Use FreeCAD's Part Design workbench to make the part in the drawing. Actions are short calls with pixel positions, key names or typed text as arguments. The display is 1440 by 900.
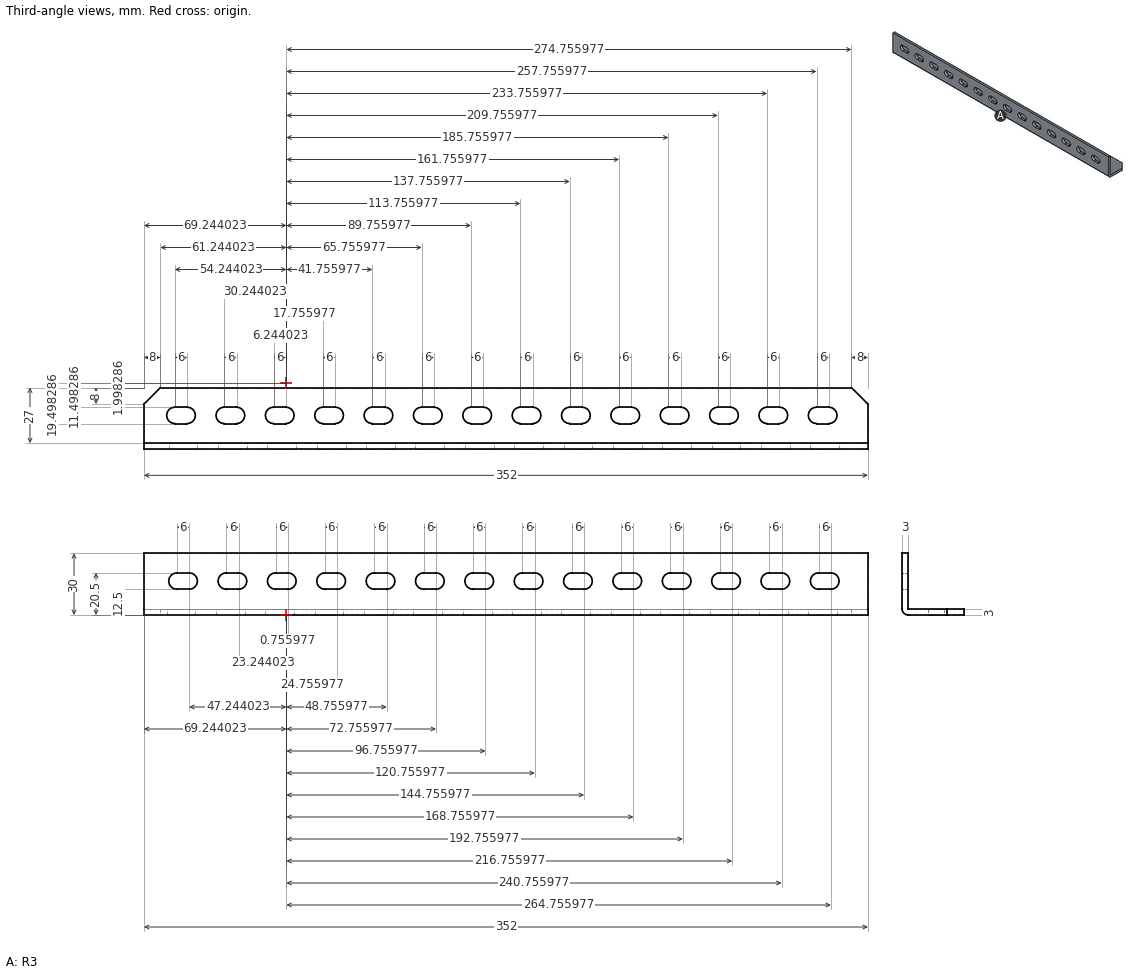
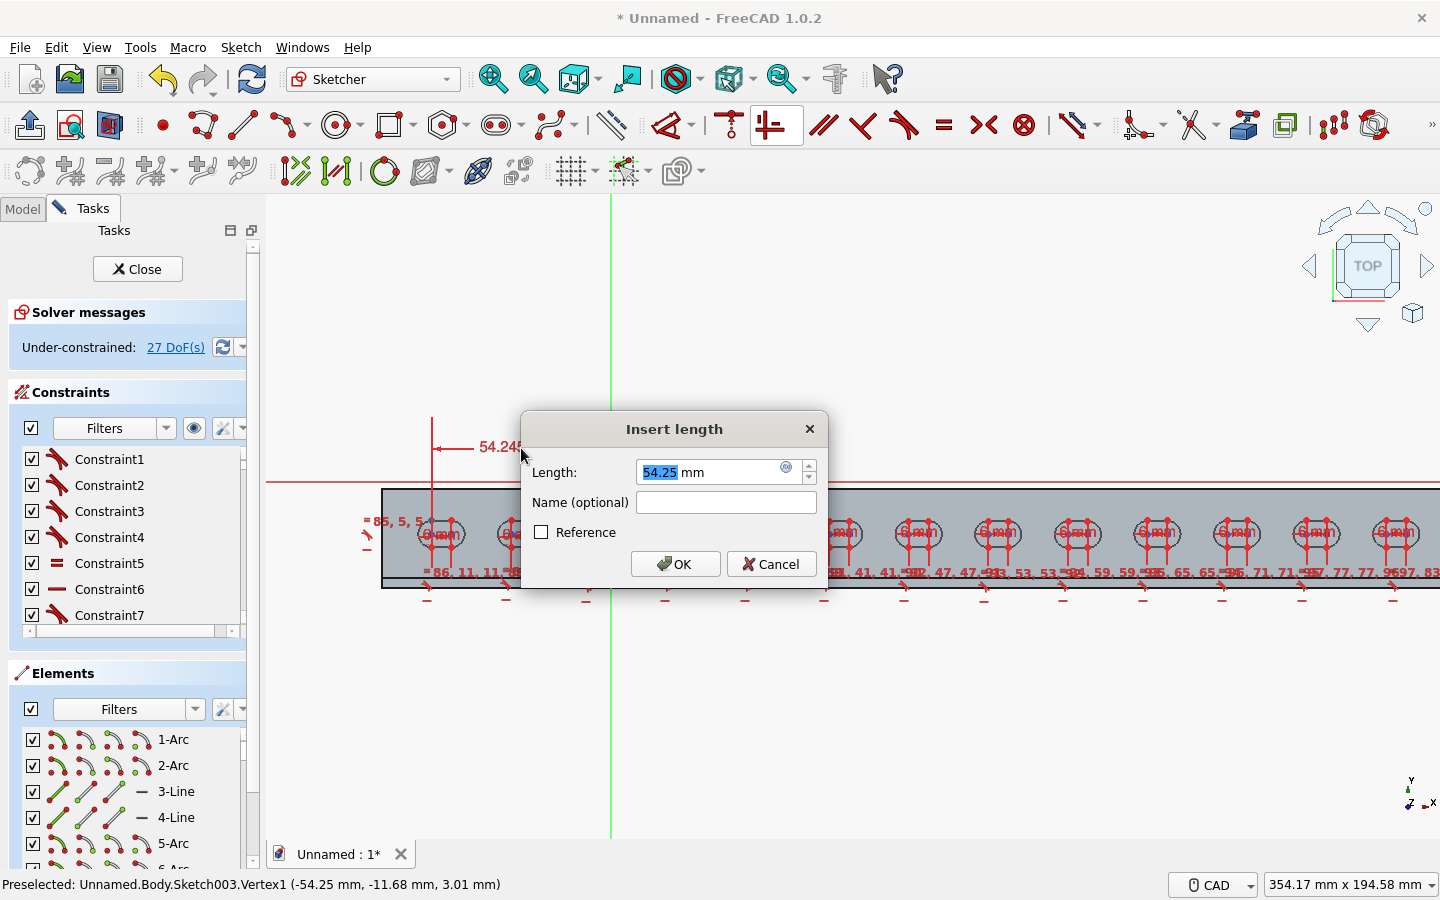
text(54.244023)
key(Return)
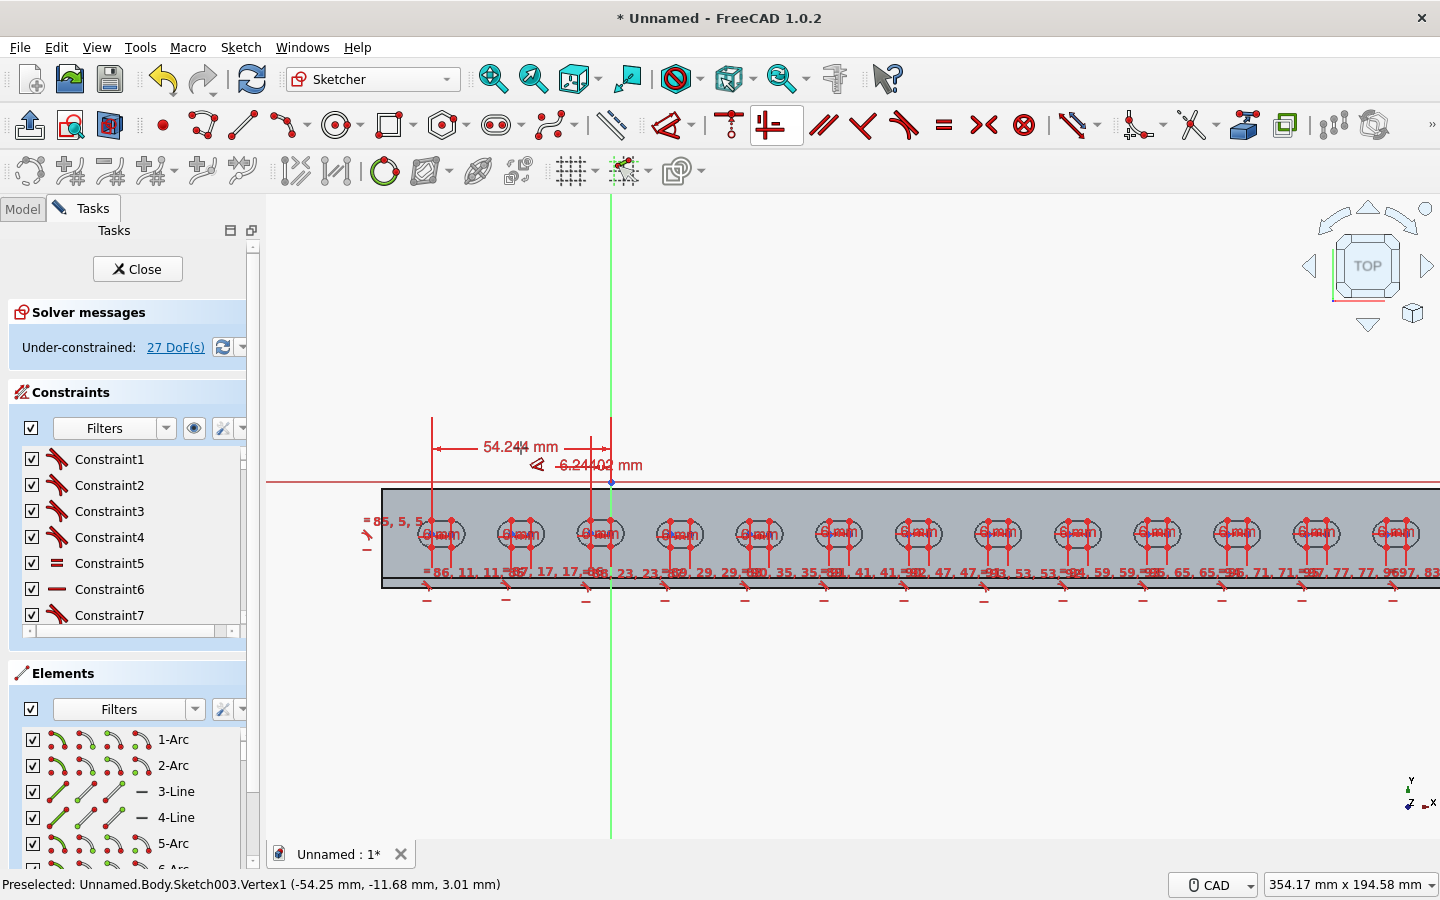
click(432, 521)
click(398, 502)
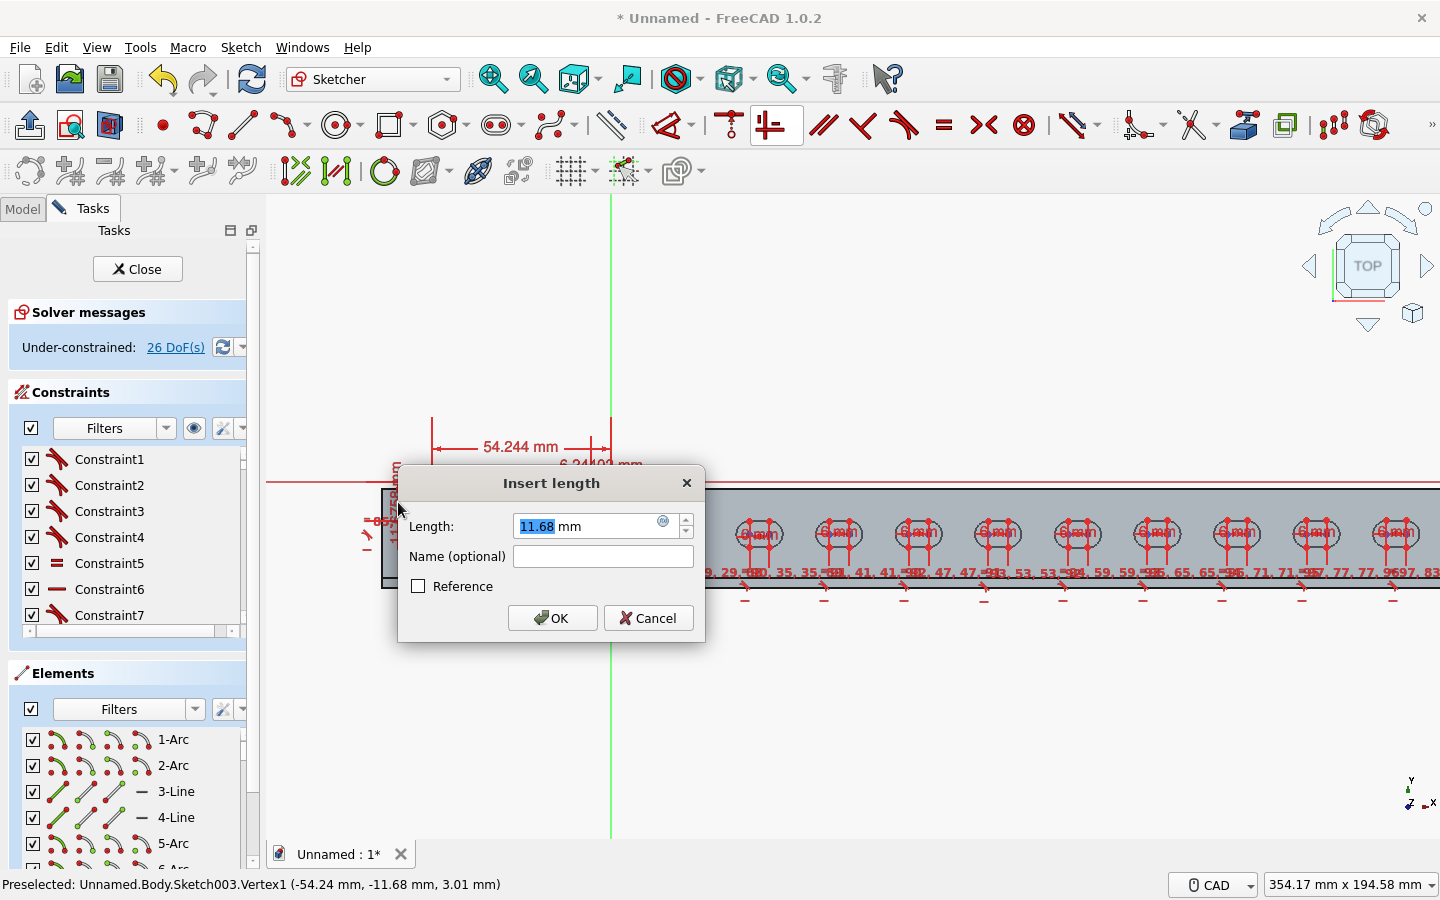
text(11.498286)
key(Return)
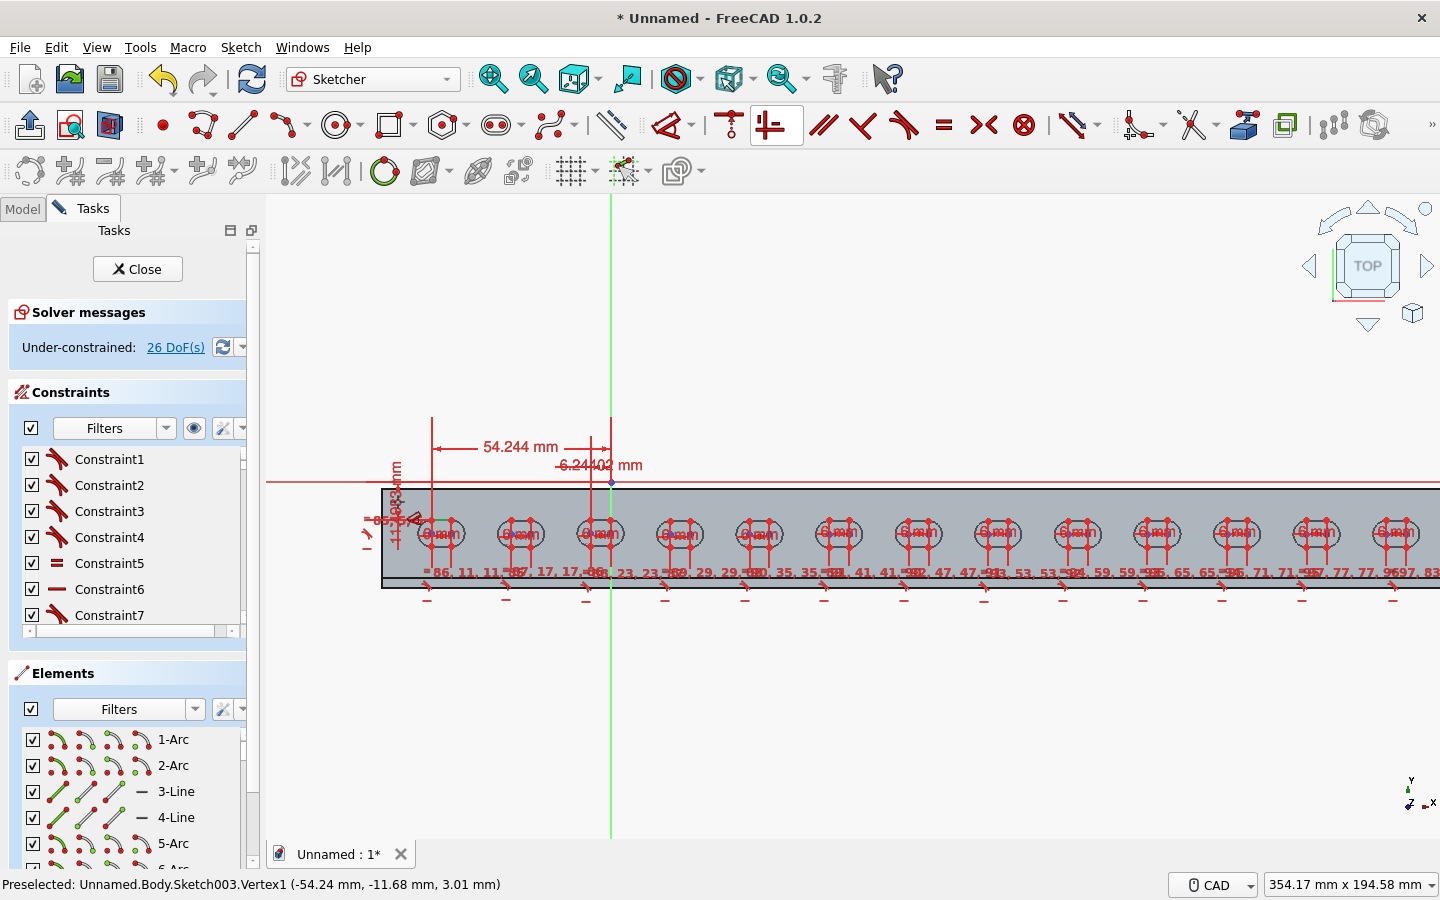
click(432, 547)
click(645, 514)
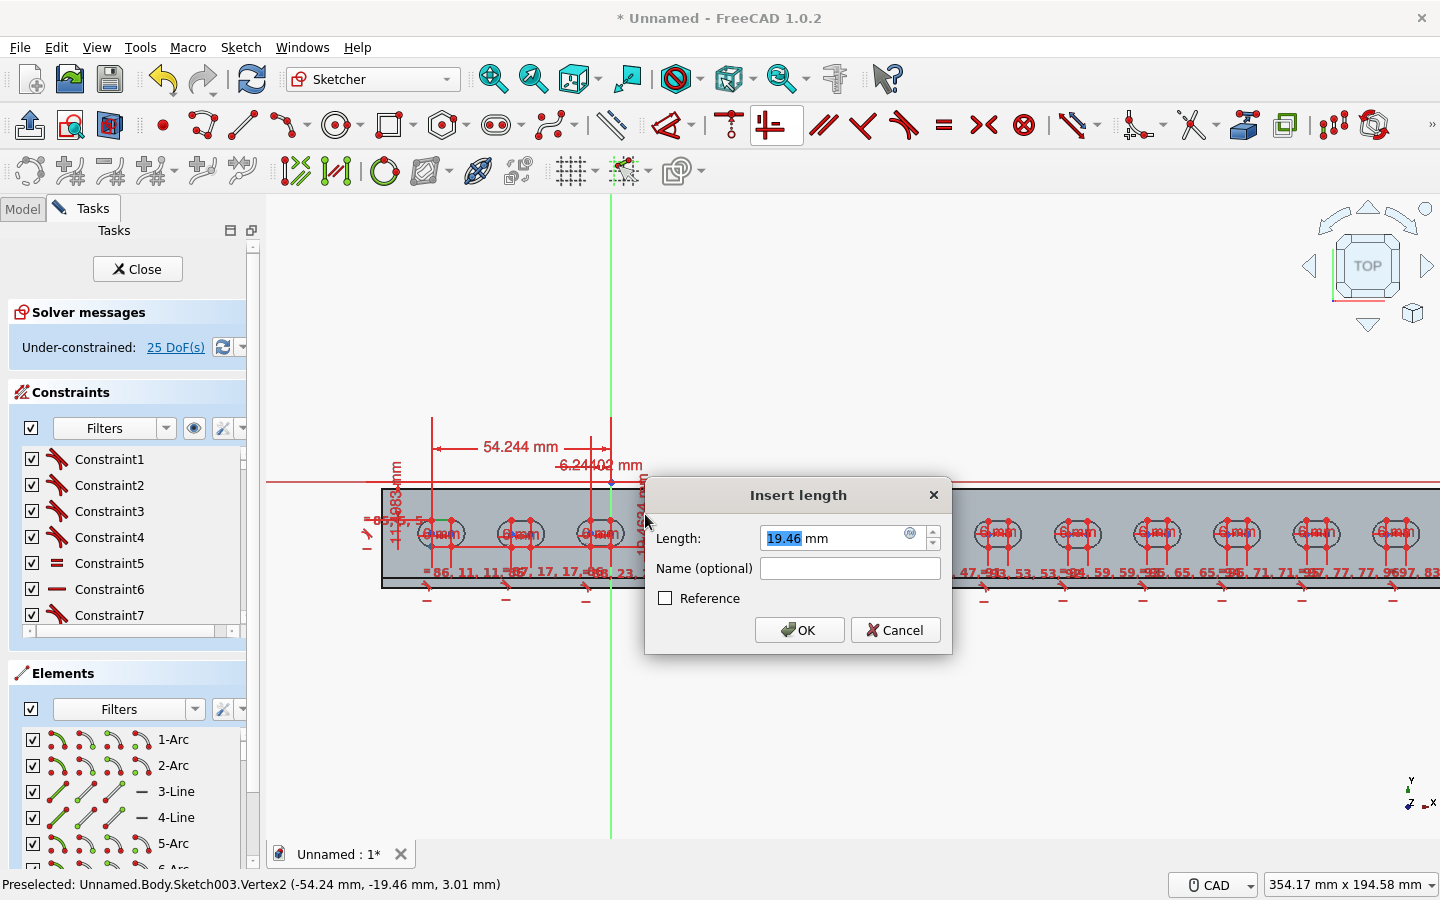
text(19.498286)
key(Return)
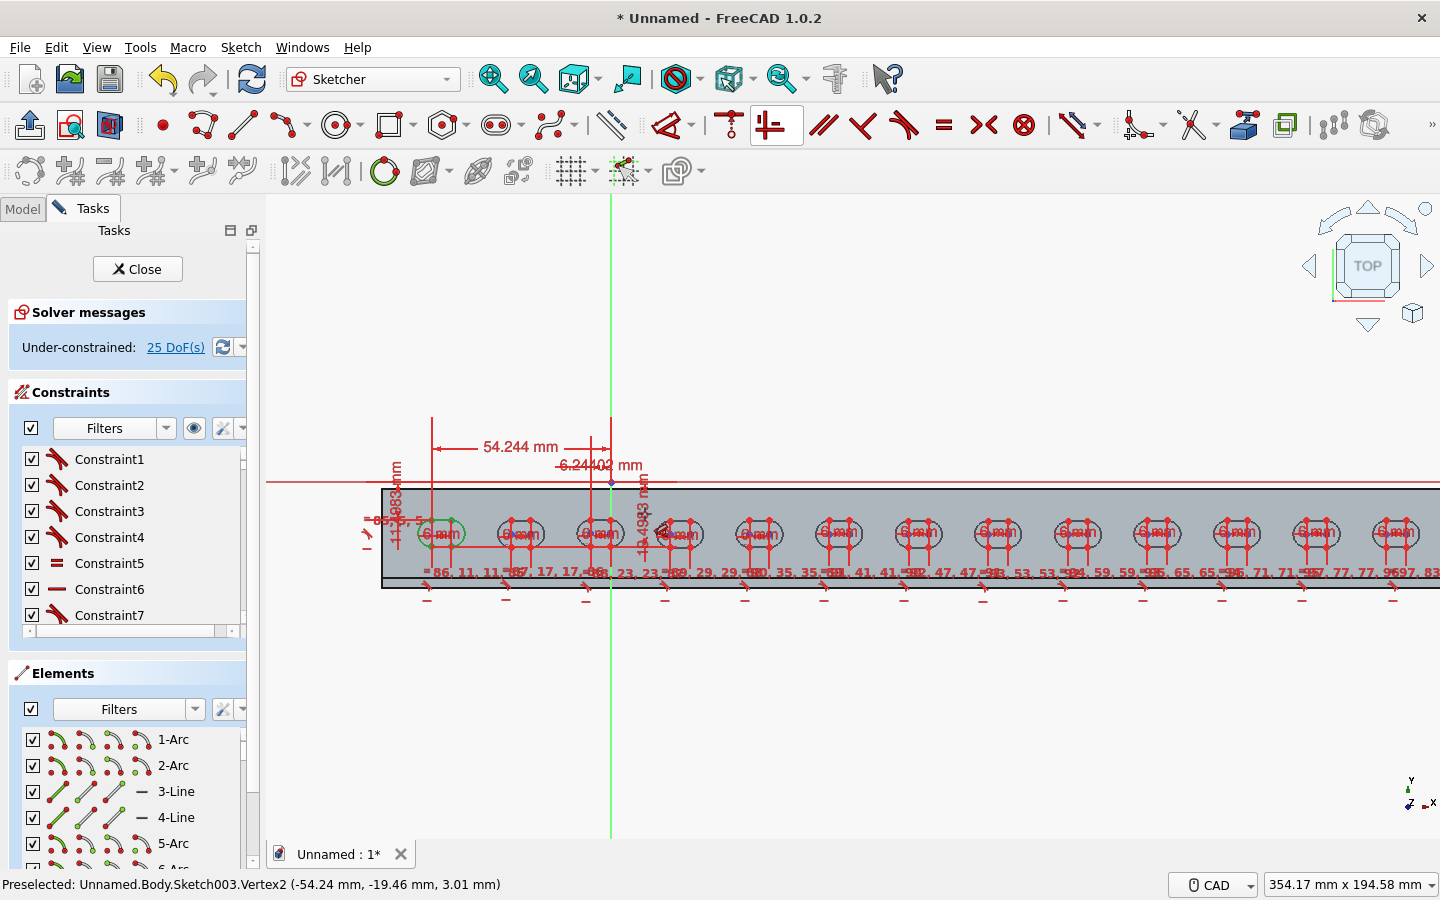
click(511, 521)
click(561, 424)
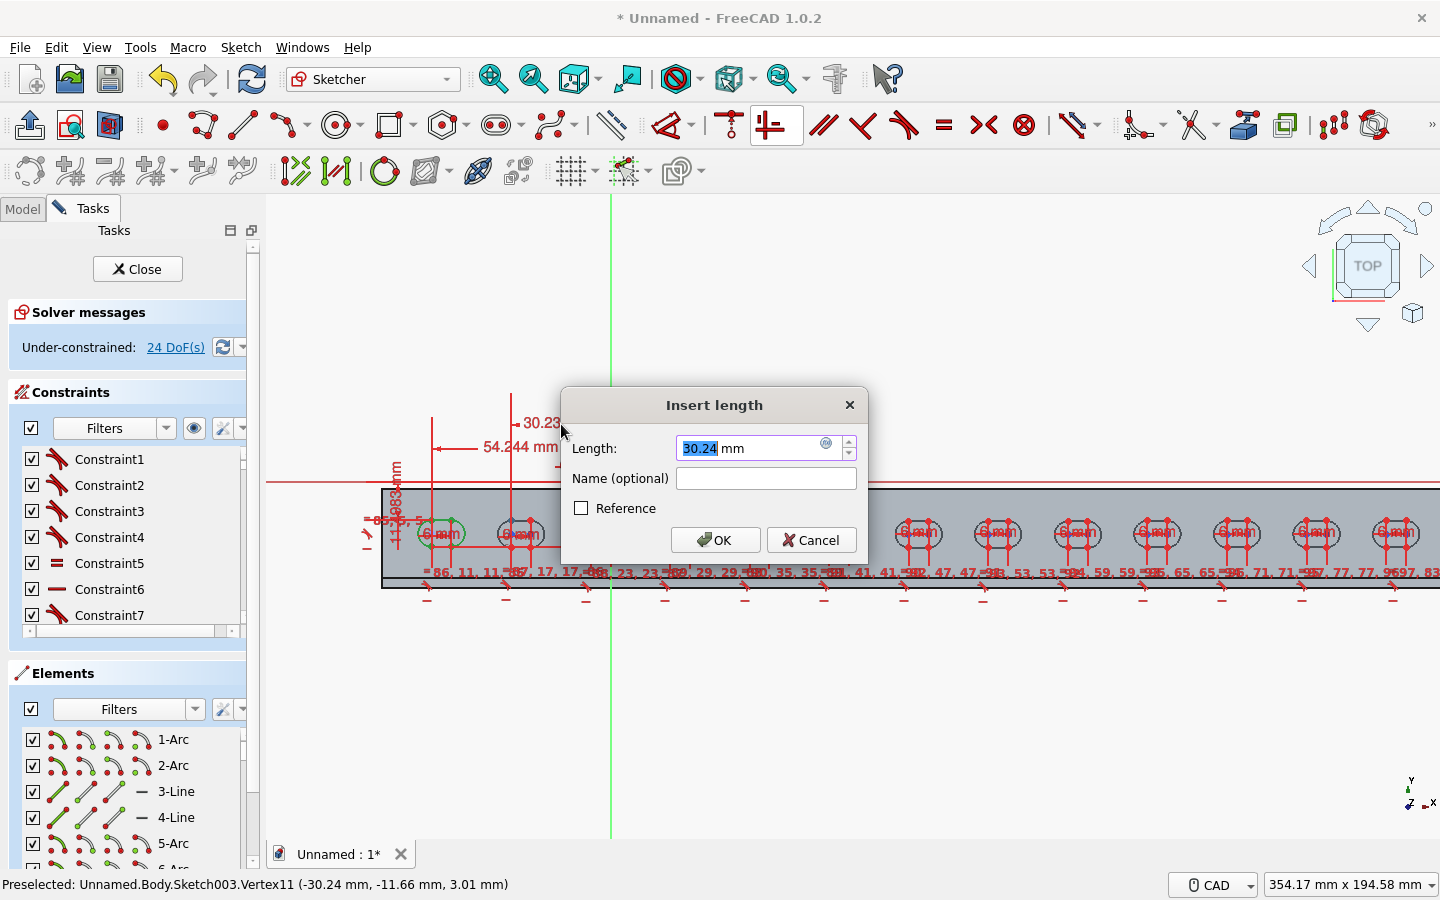
text(30.244023)
key(Return)